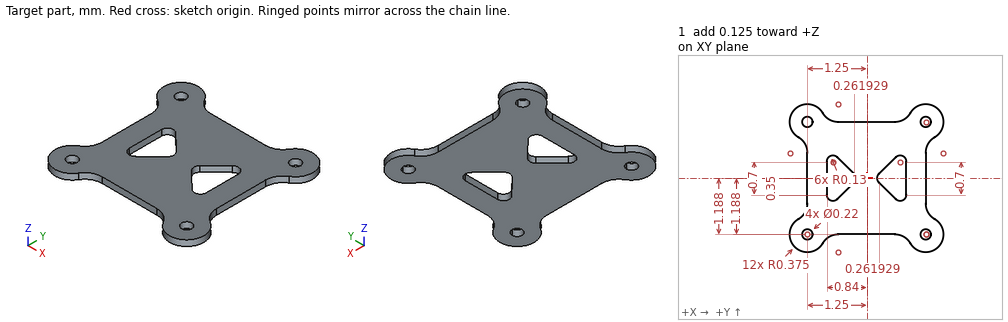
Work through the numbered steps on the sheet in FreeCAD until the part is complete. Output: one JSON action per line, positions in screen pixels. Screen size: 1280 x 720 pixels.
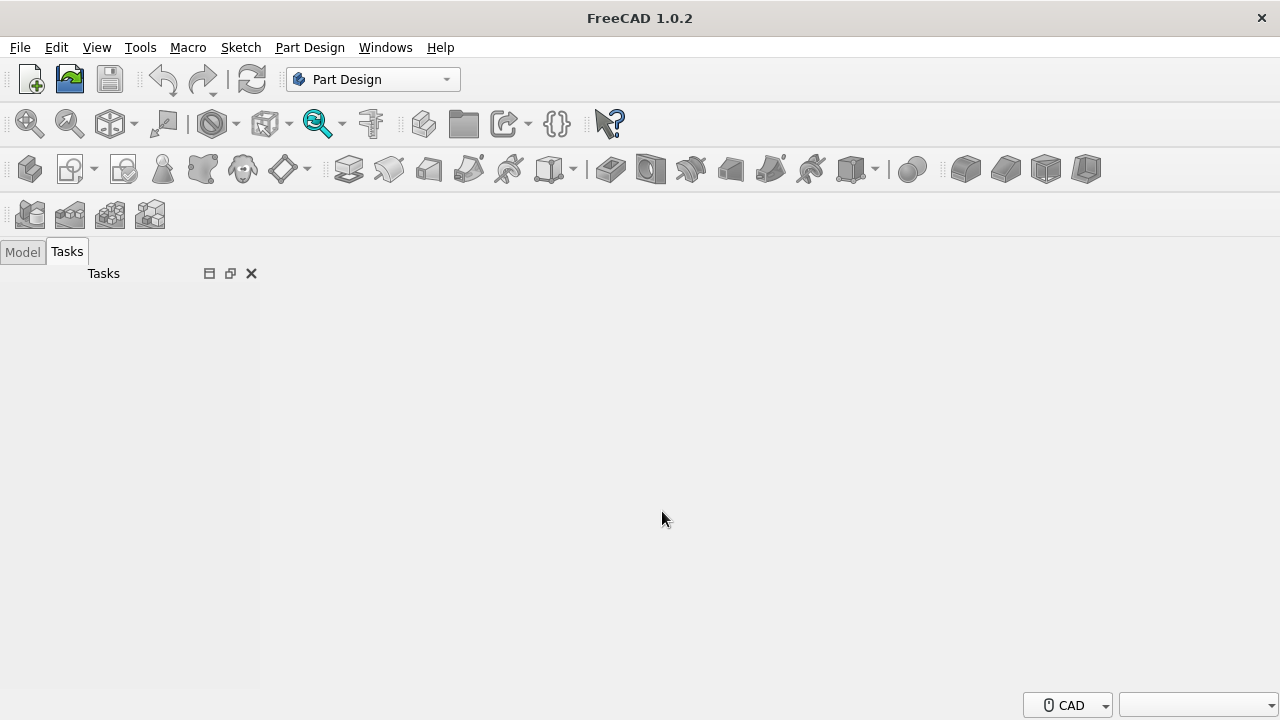
{"action": "left_click", "coordinate": [30, 80]}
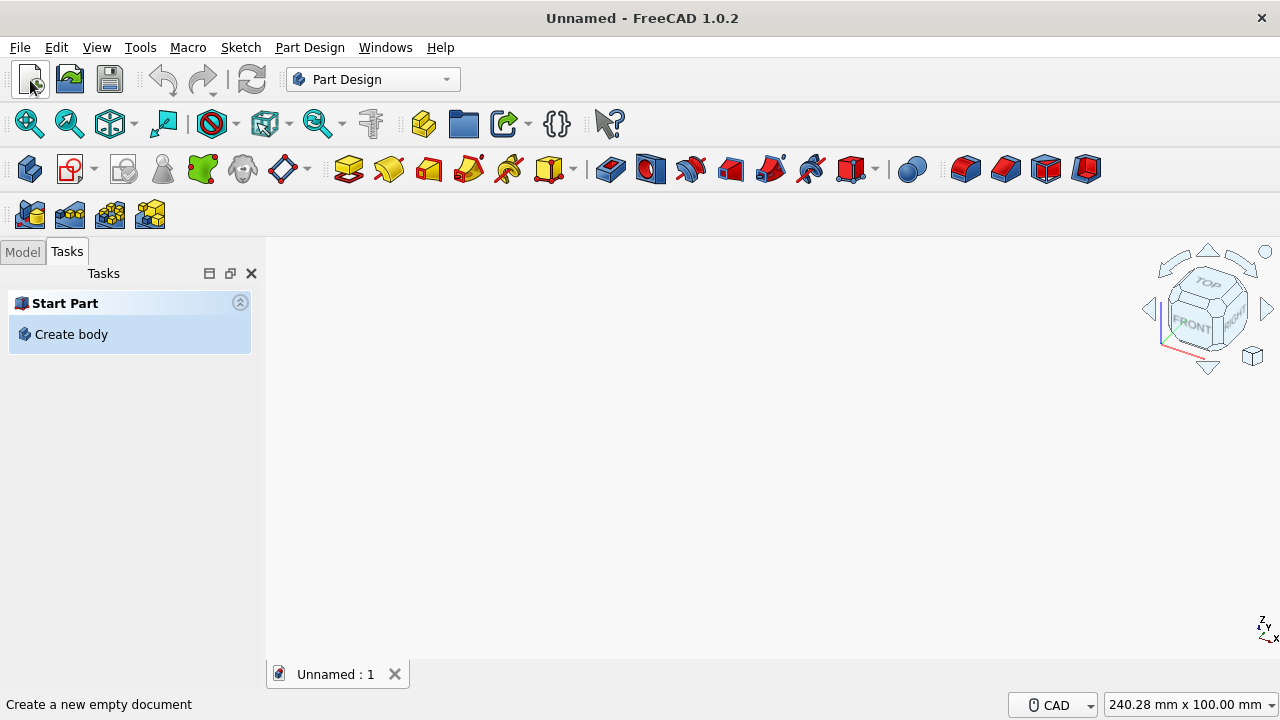
{"action": "left_click", "coordinate": [70, 170]}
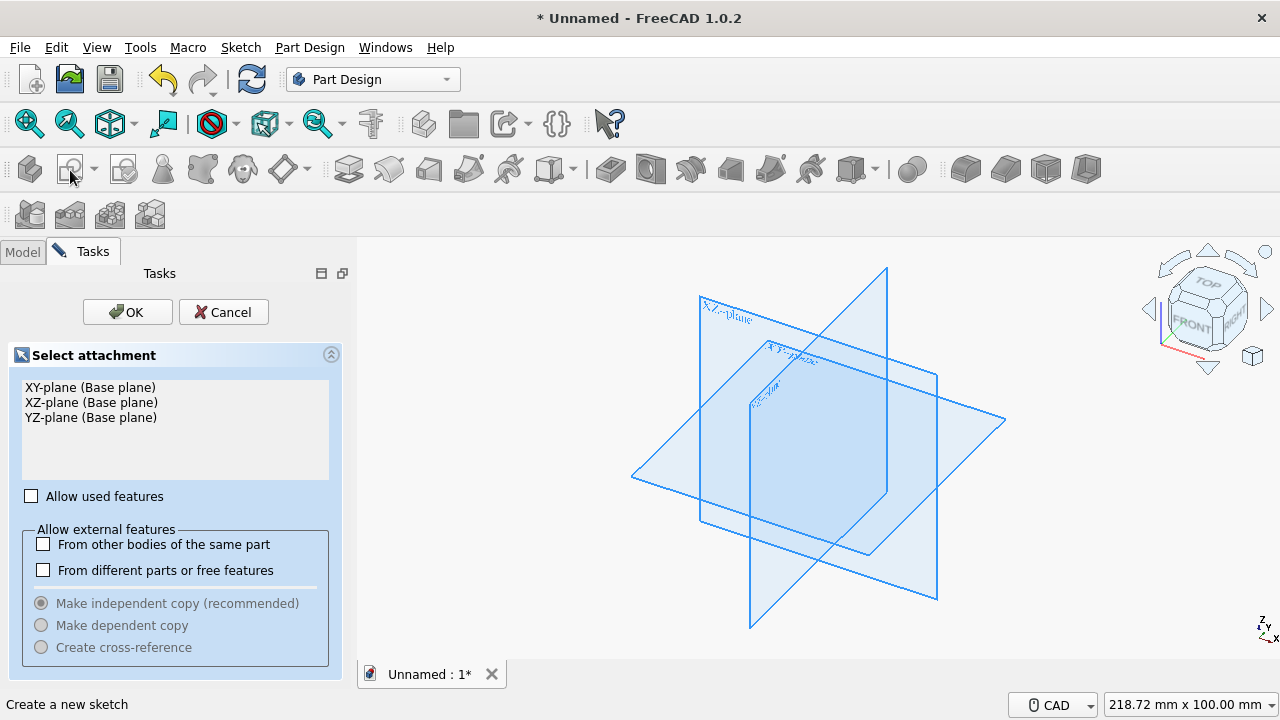
{"action": "left_click", "coordinate": [82, 388]}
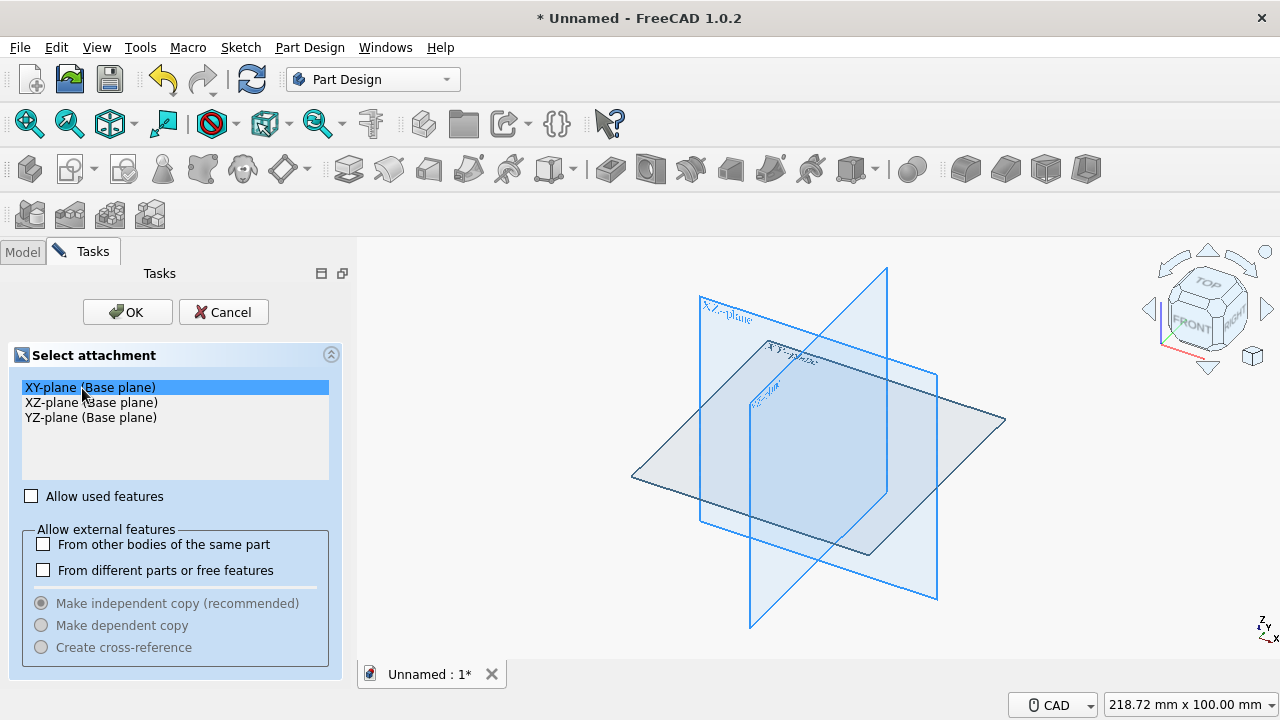
{"action": "left_click", "coordinate": [128, 312]}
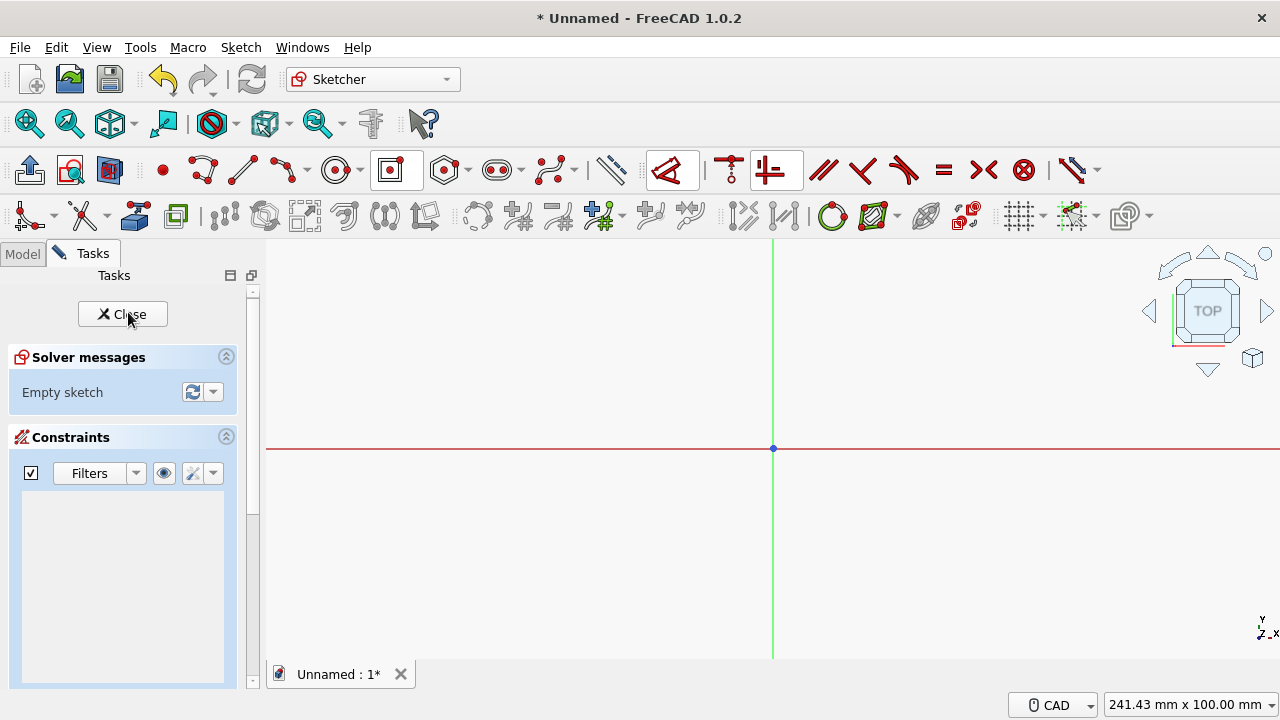
{"action": "scroll", "coordinate": [777, 449], "scroll_direction": "up", "scroll_amount": 15}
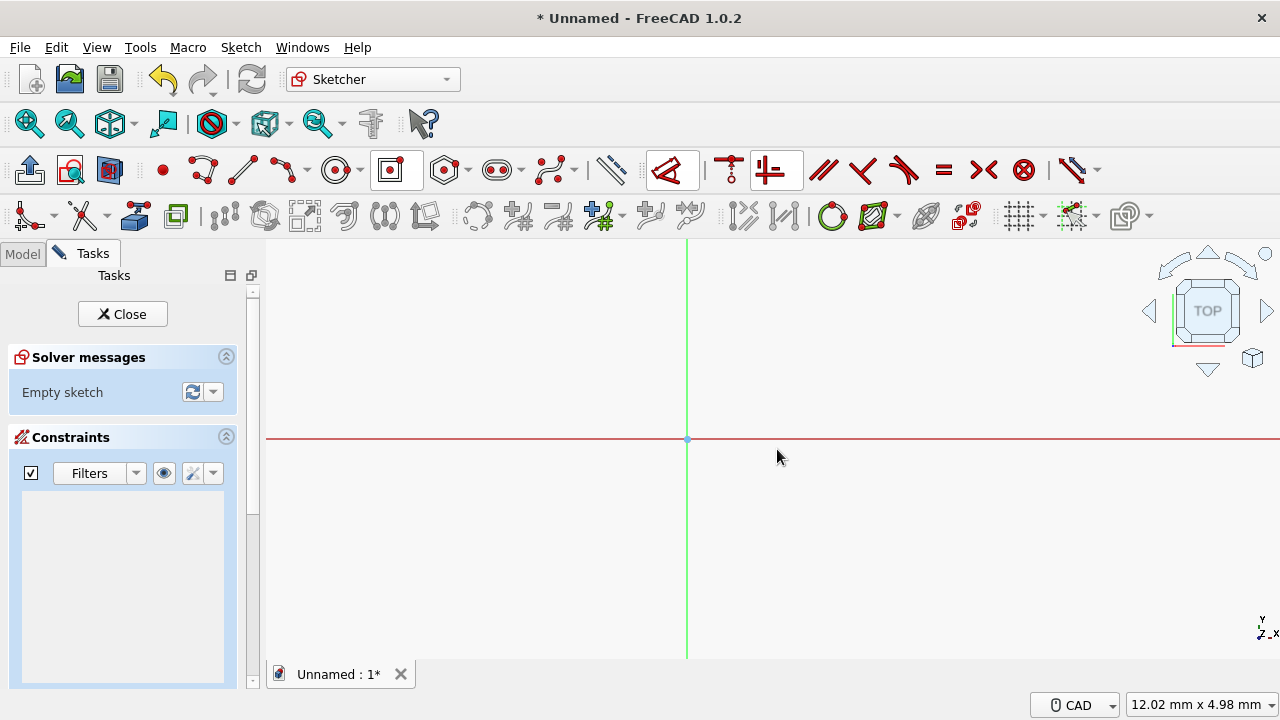
{"action": "left_click", "coordinate": [244, 170]}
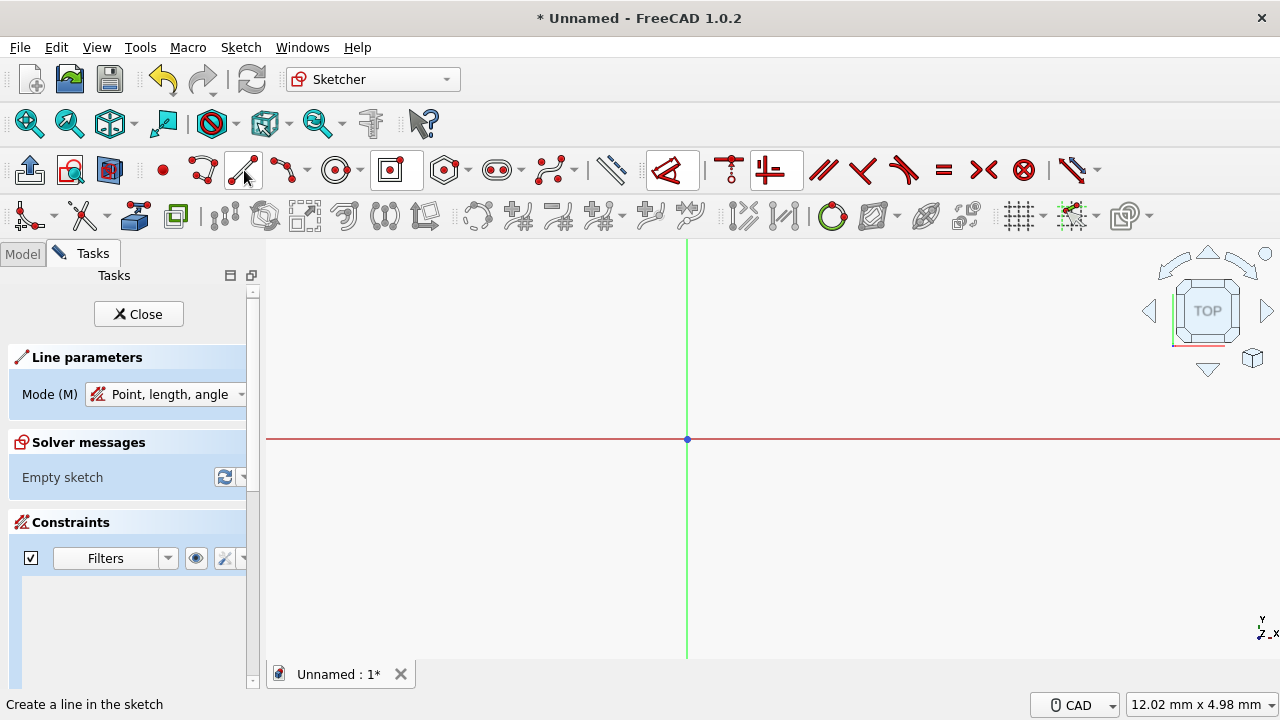
{"action": "left_click", "coordinate": [582, 394]}
{"action": "left_click", "coordinate": [582, 485]}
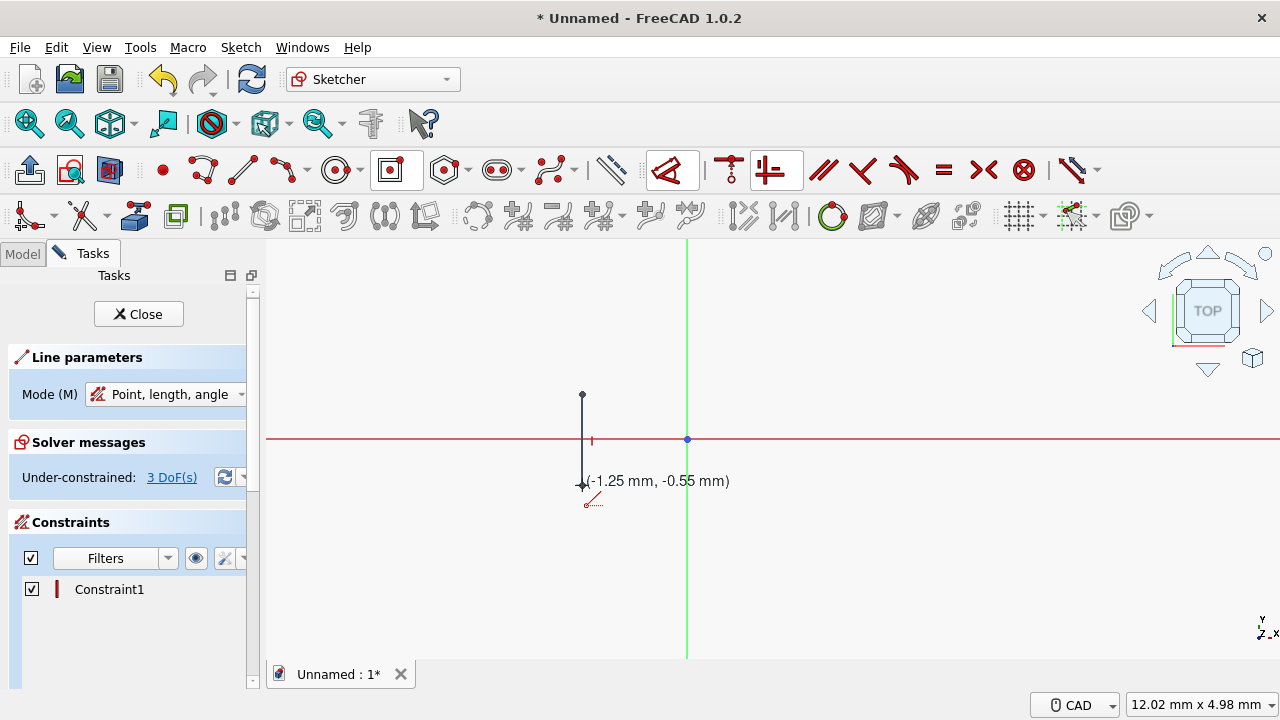
{"action": "left_click", "coordinate": [636, 540]}
{"action": "left_click", "coordinate": [738, 540]}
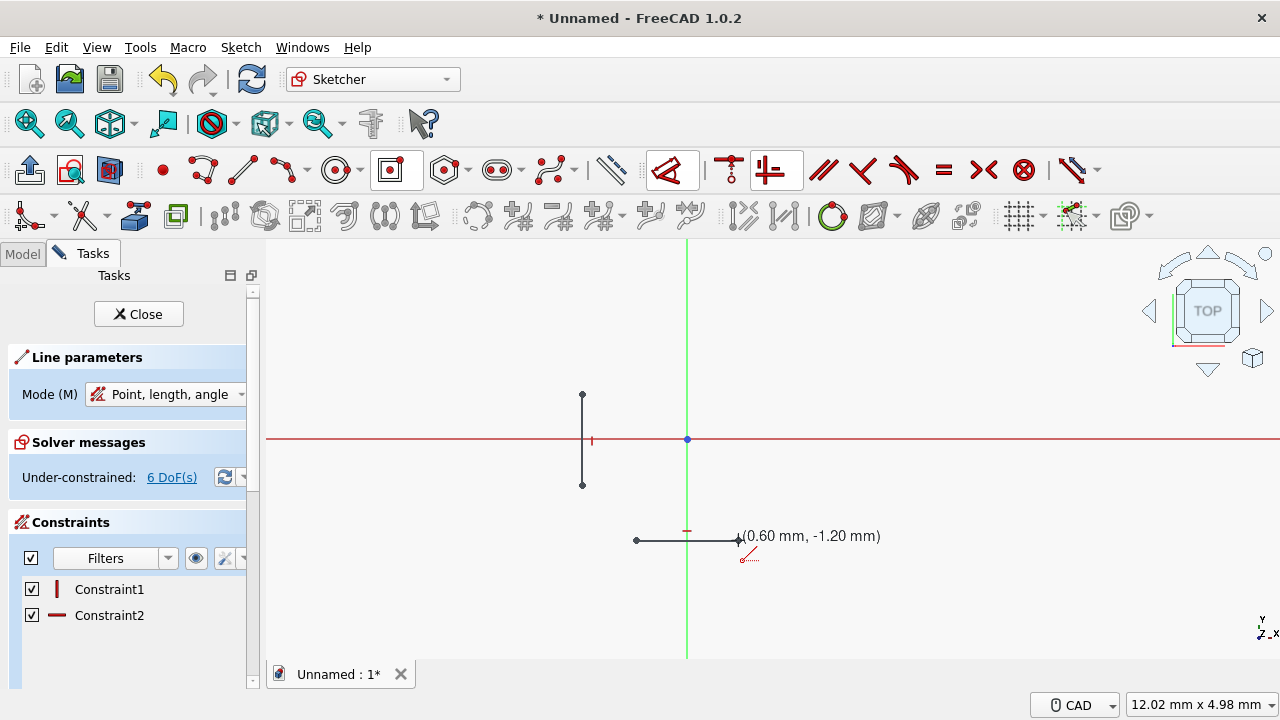
{"action": "left_click", "coordinate": [792, 485]}
{"action": "left_click", "coordinate": [792, 394]}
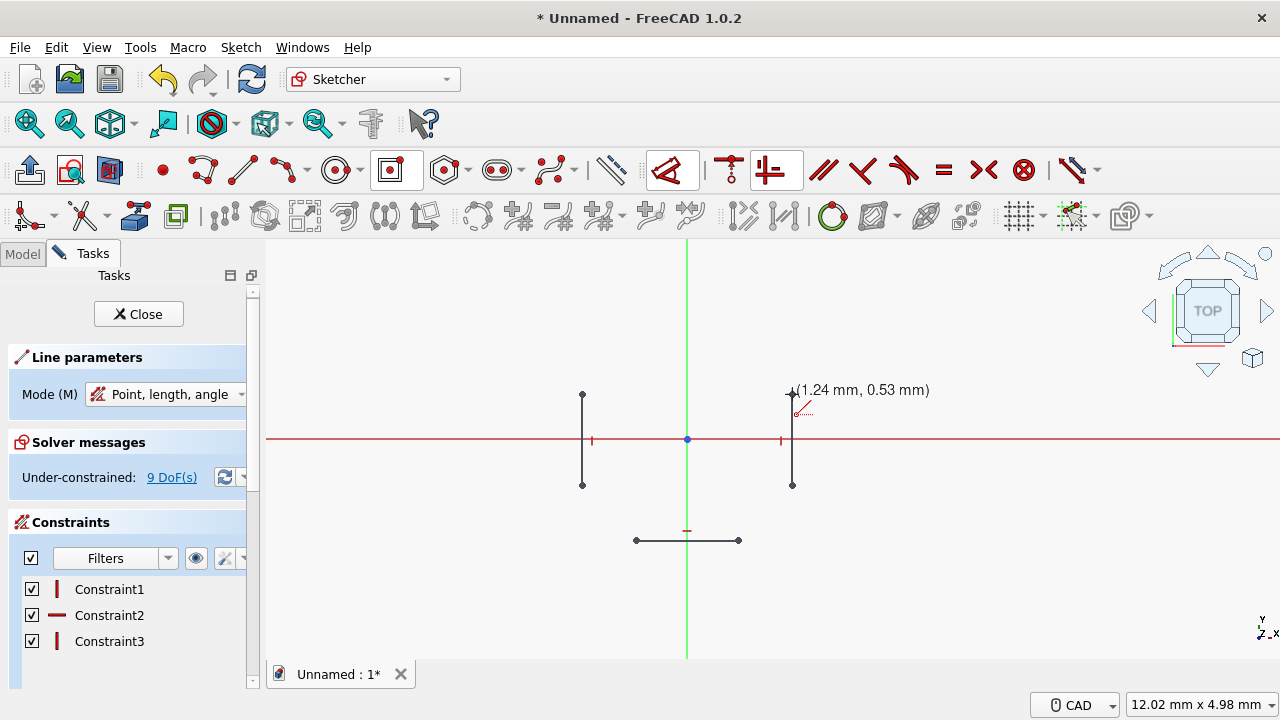
{"action": "left_click", "coordinate": [738, 339]}
{"action": "left_click", "coordinate": [636, 339]}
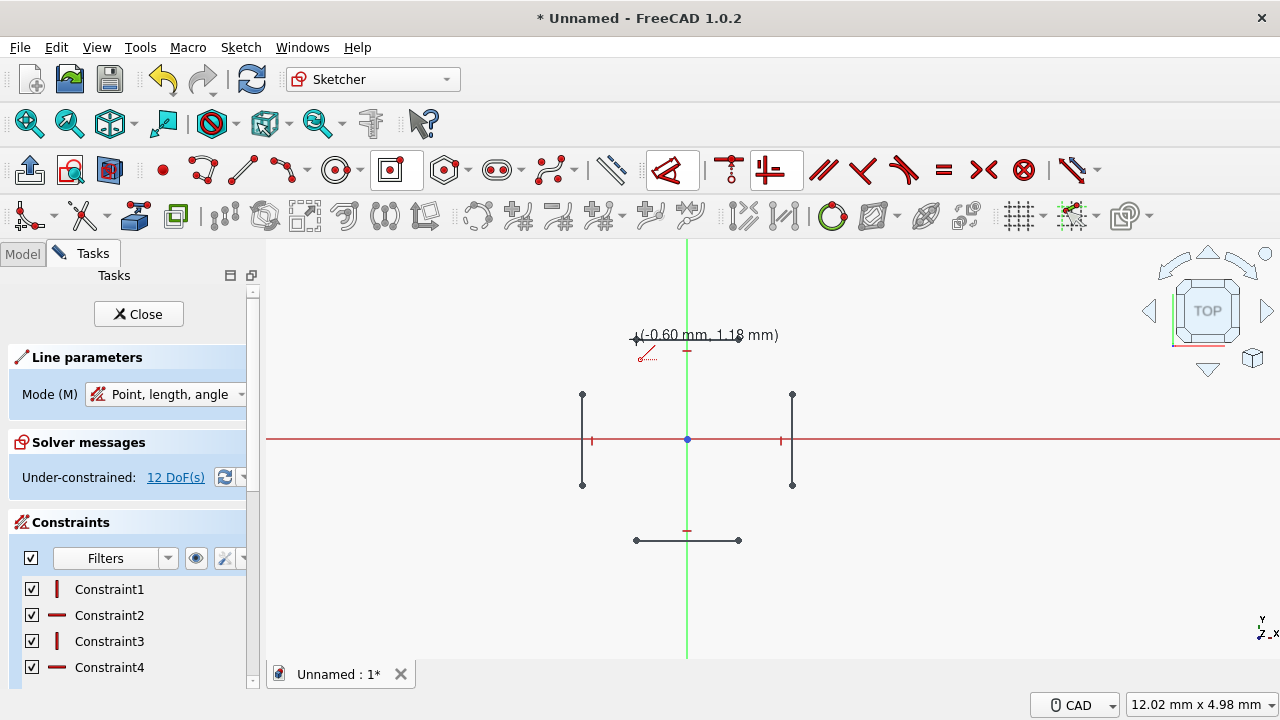
{"action": "left_click", "coordinate": [284, 170]}